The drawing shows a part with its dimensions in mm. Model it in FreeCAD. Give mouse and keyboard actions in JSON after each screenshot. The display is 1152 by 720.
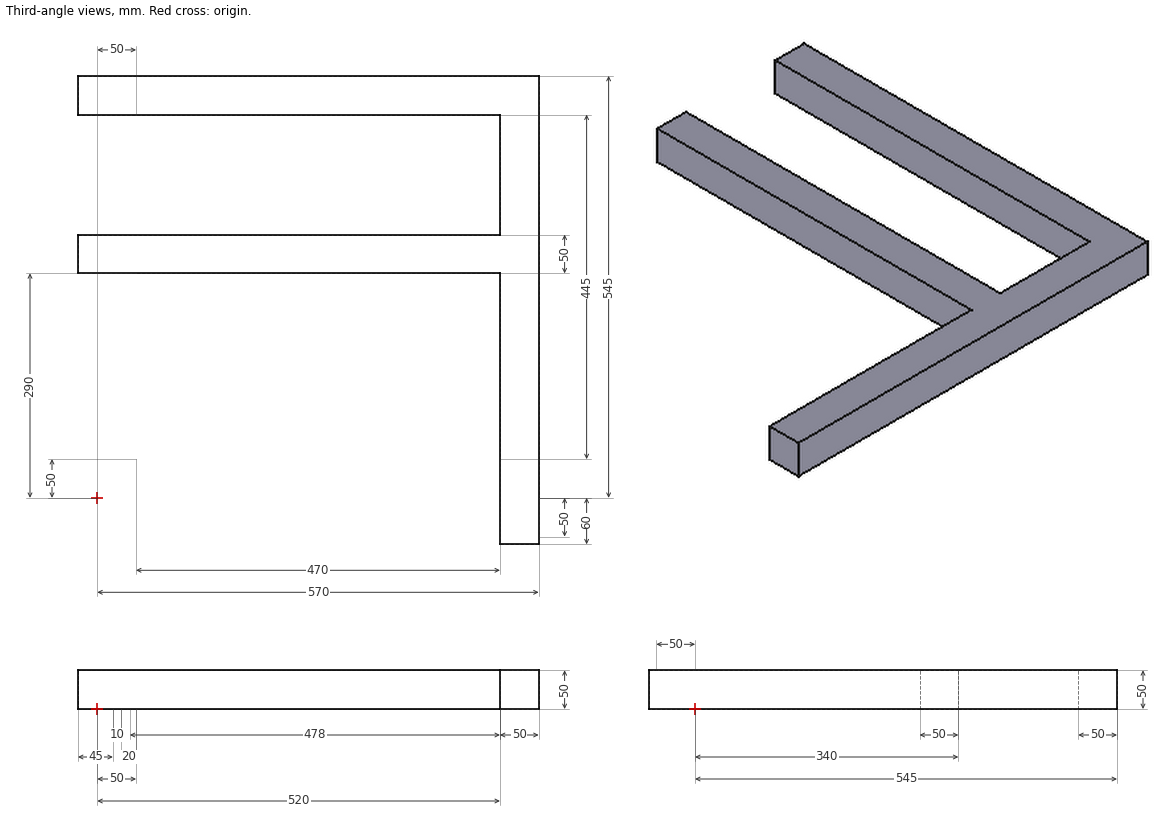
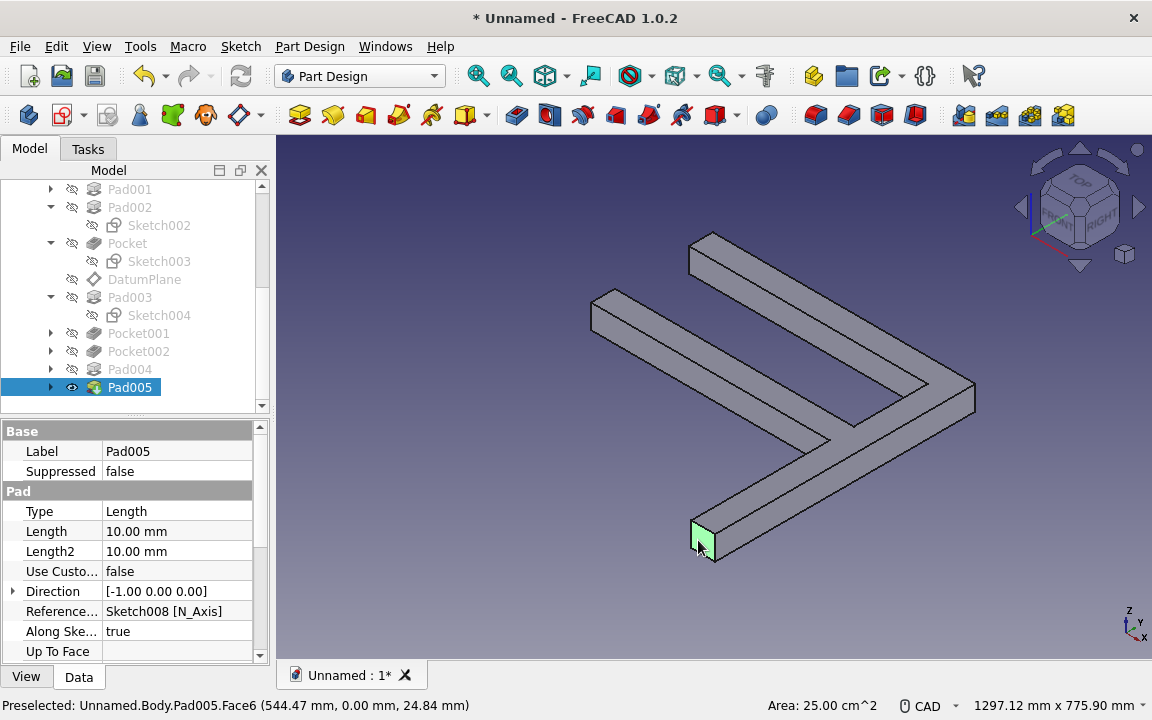
{"action": "left_click", "coordinate": [62, 116]}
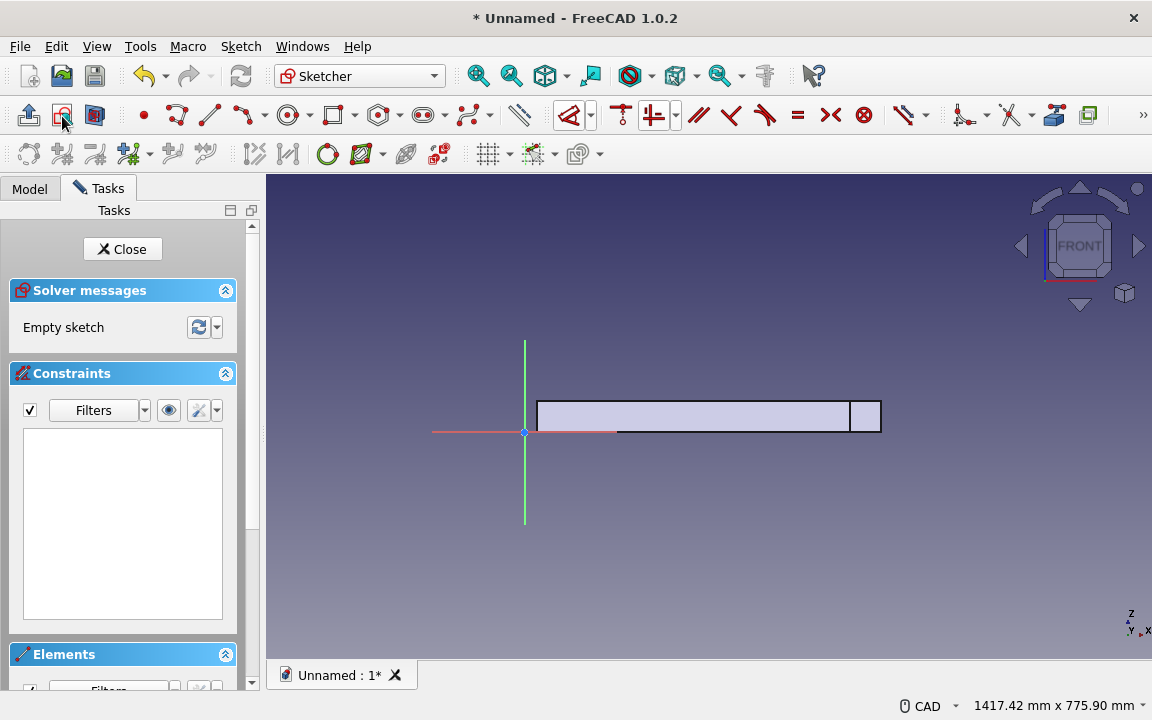
{"action": "scroll", "coordinate": [893, 416], "scroll_direction": "up", "scroll_amount": 11}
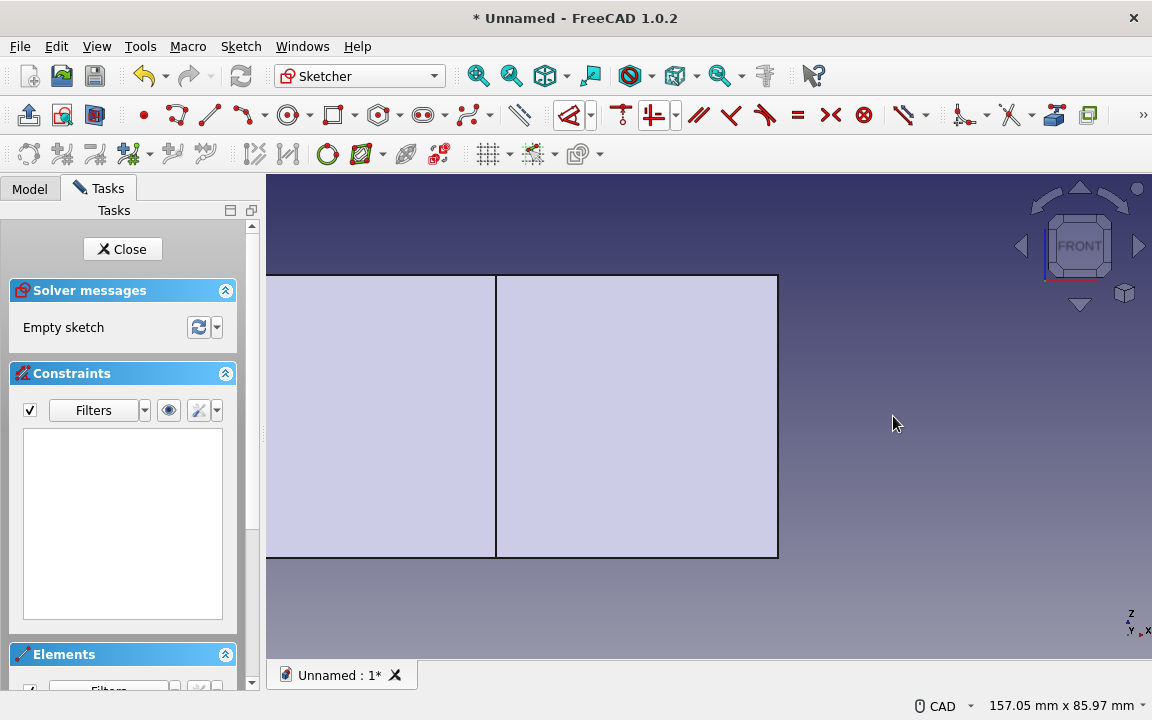
{"action": "key", "text": "g r"}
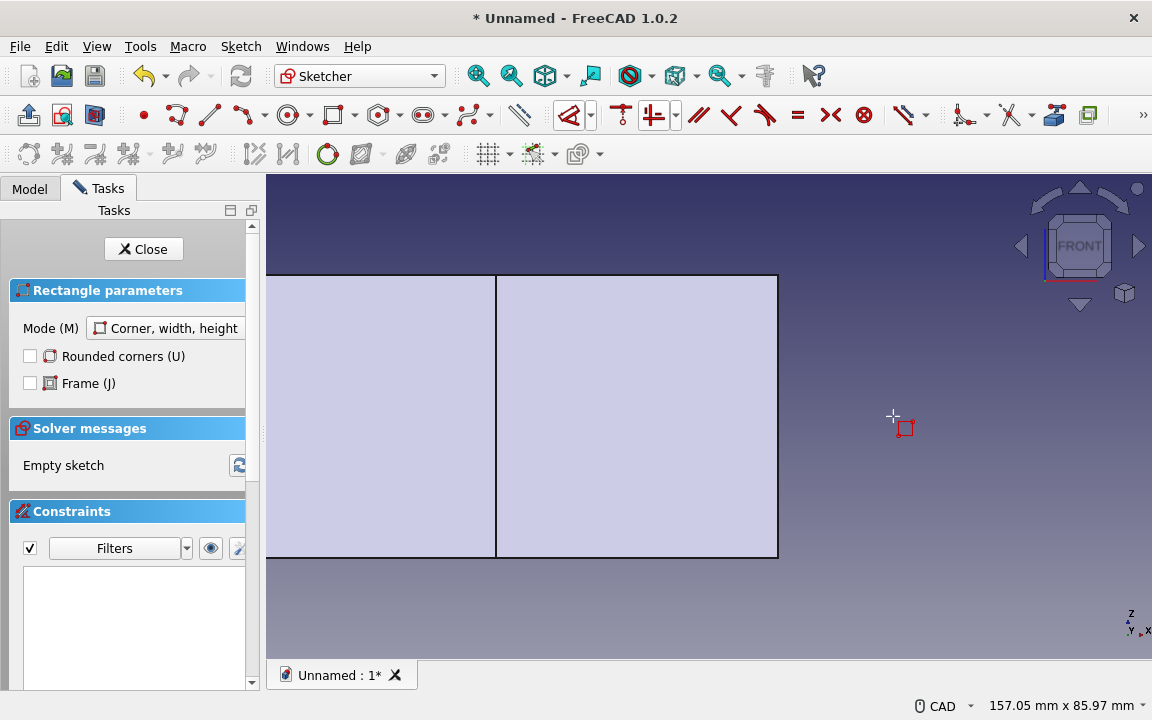
{"action": "left_click", "coordinate": [496, 275]}
{"action": "left_click", "coordinate": [778, 558]}
{"action": "key", "text": "Escape"}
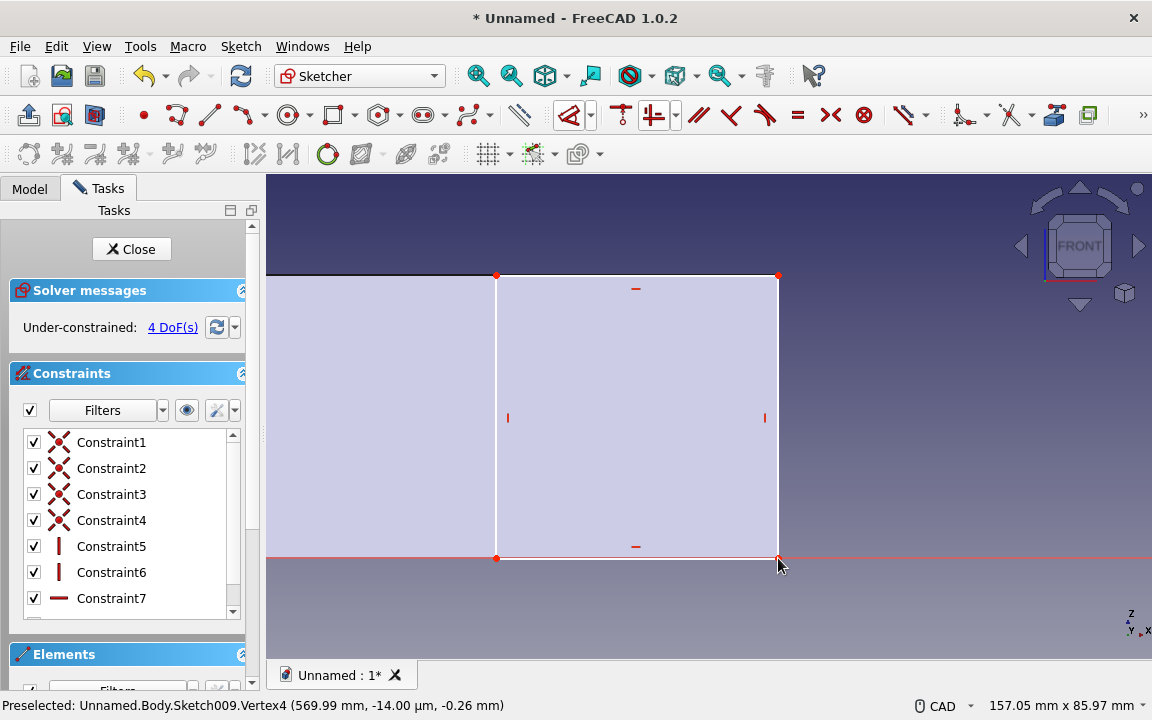
{"action": "left_click", "coordinate": [496, 559]}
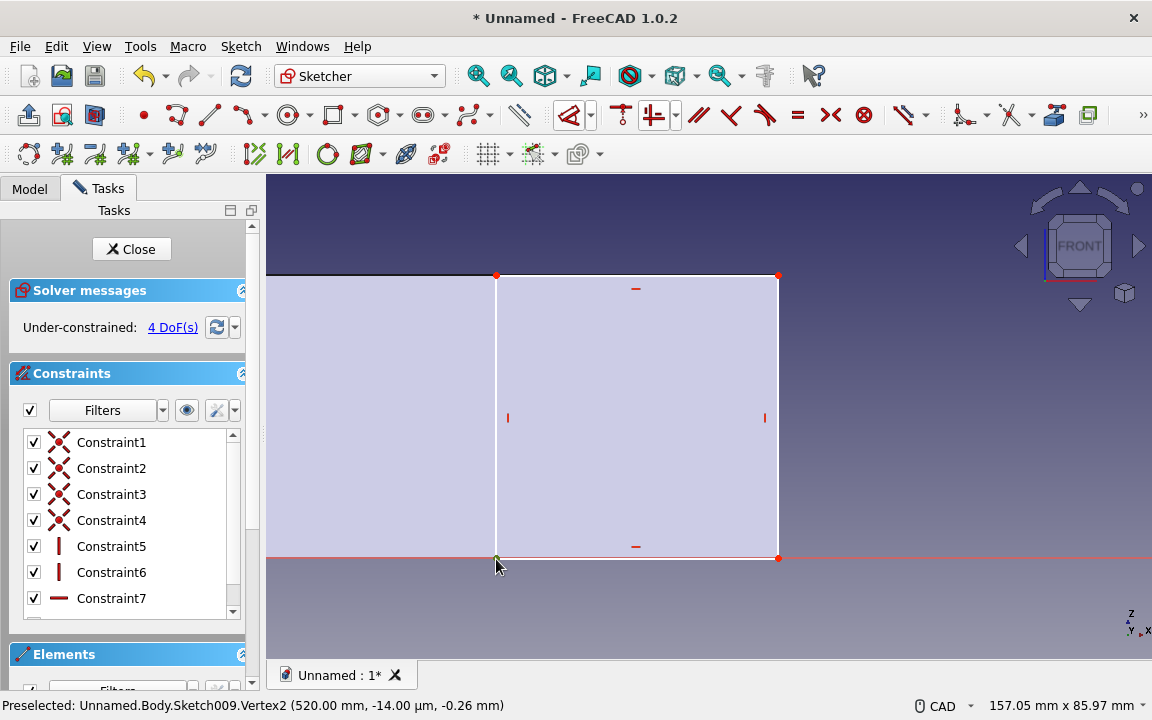
{"action": "left_click", "coordinate": [344, 558]}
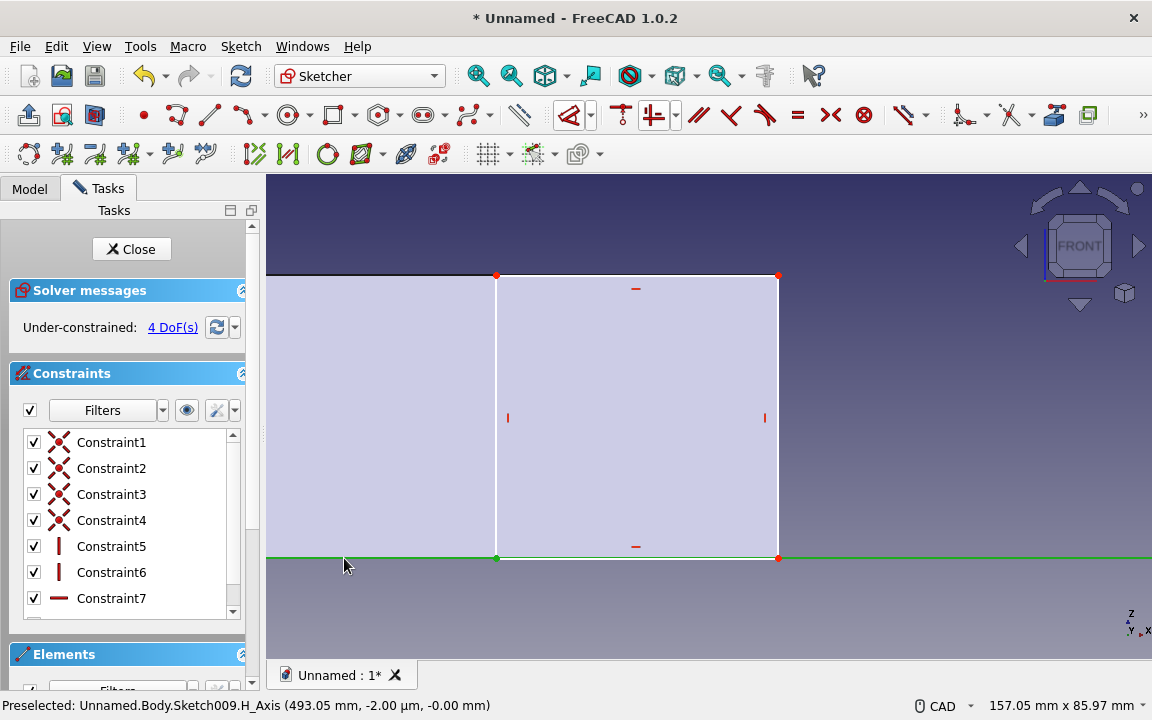
{"action": "key", "text": "c"}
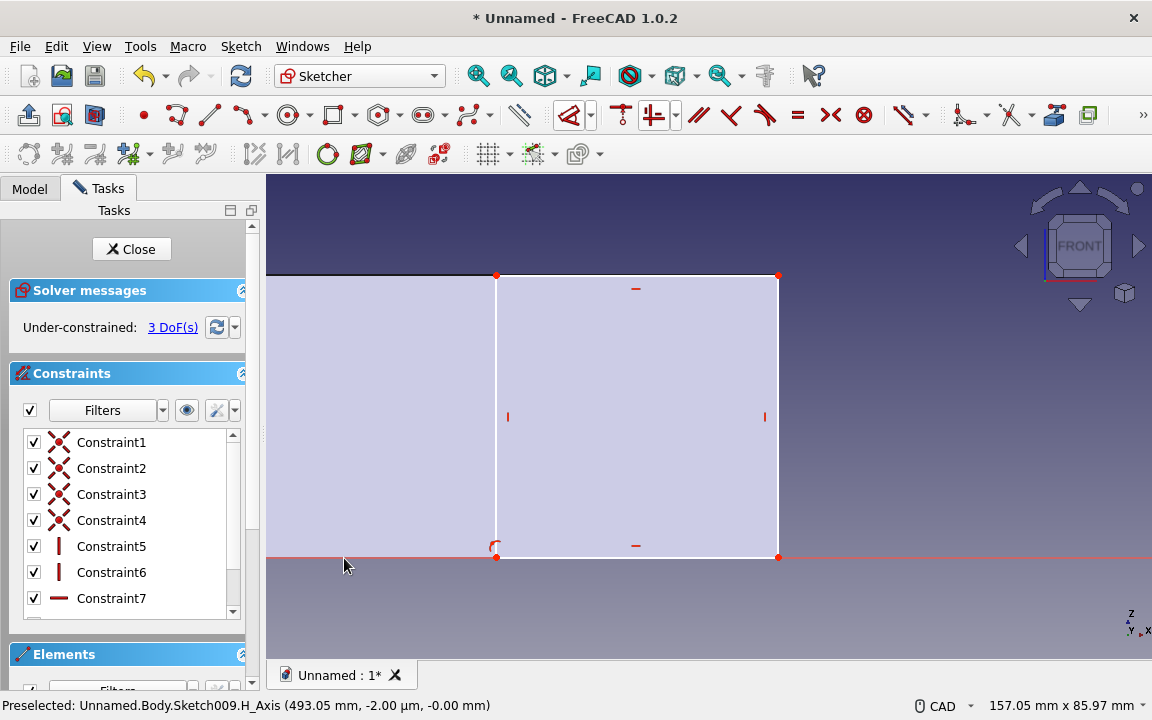
{"action": "left_click", "coordinate": [496, 360]}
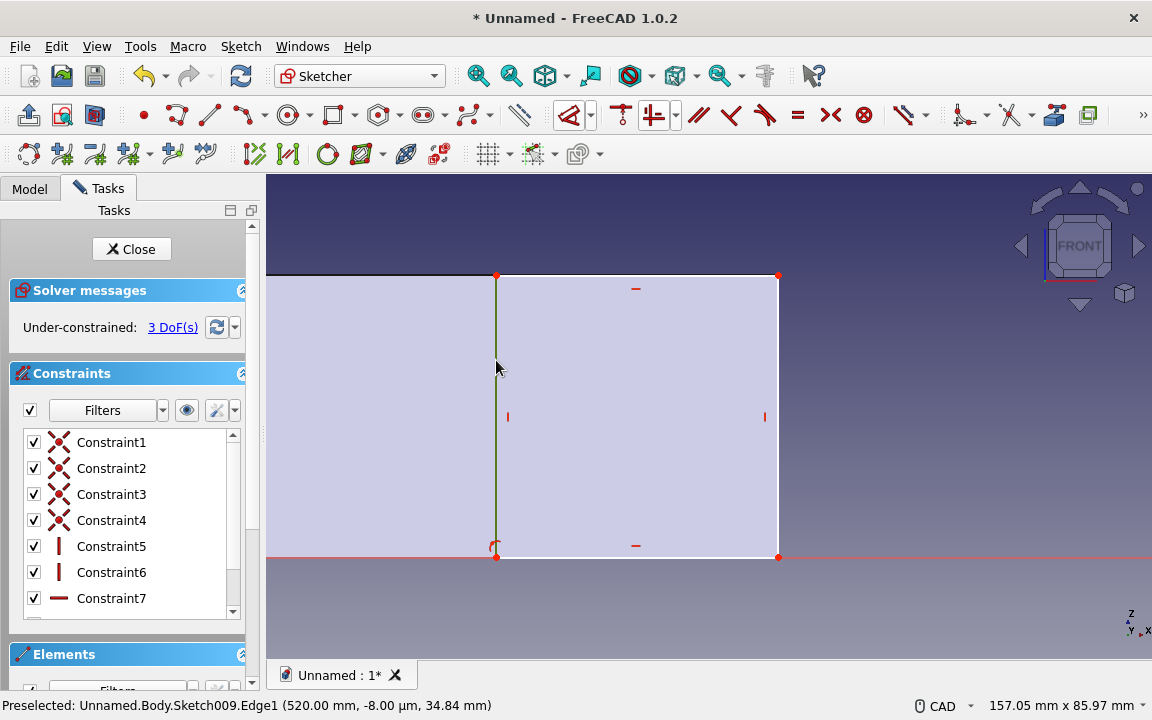
{"action": "key", "text": "i"}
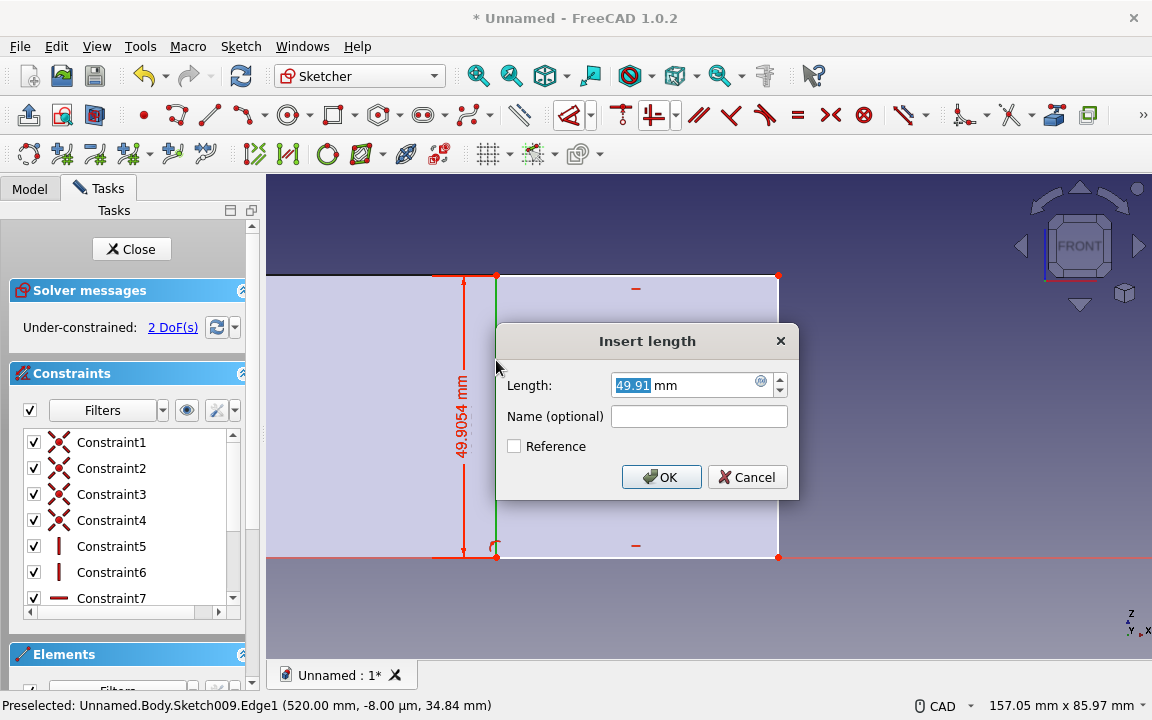
{"action": "type", "text": "50"}
{"action": "key", "text": "Return"}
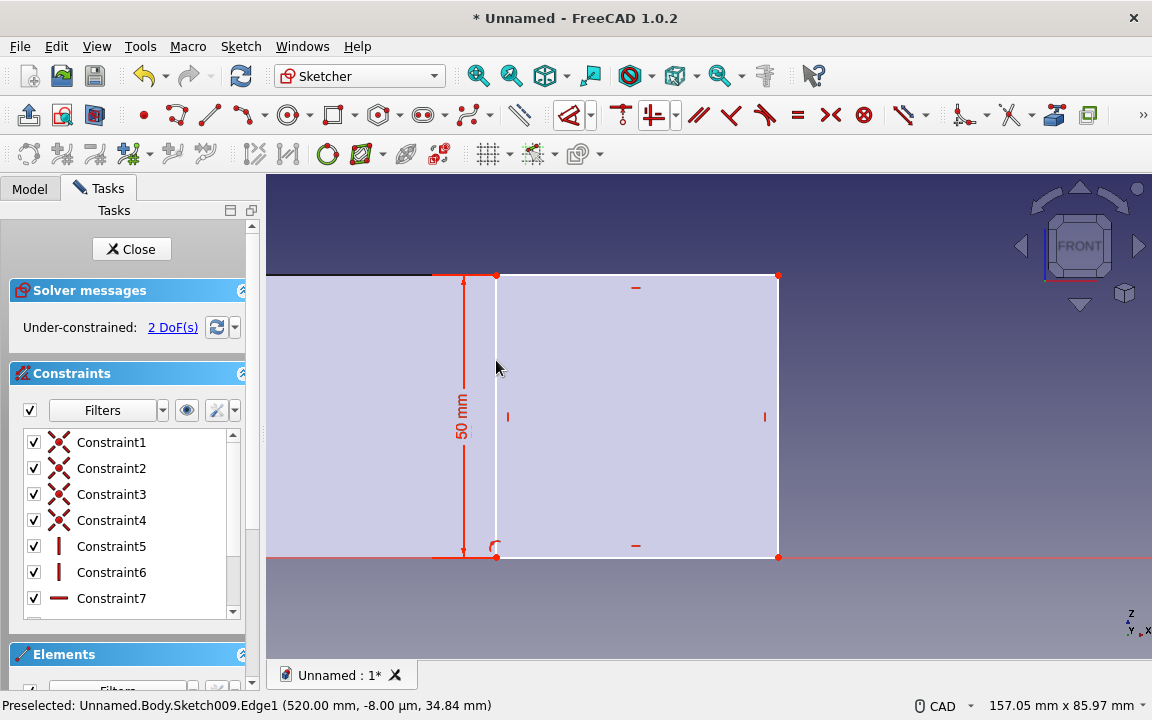
{"action": "left_click", "coordinate": [581, 558]}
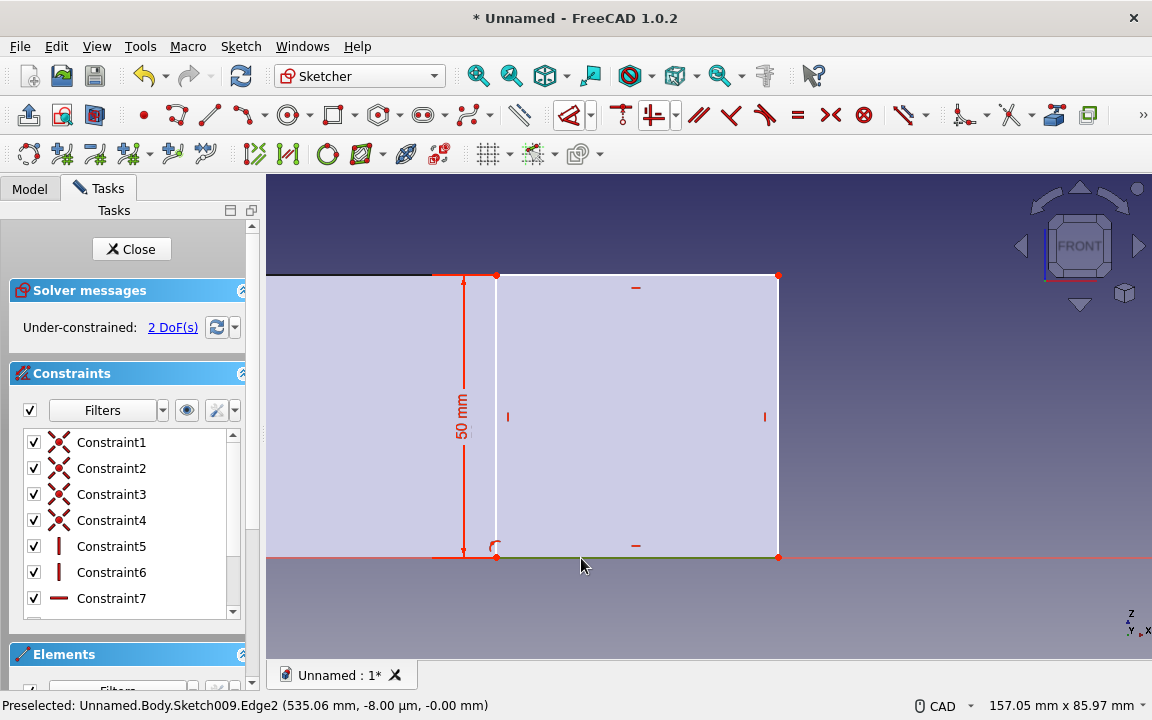
{"action": "left_click", "coordinate": [590, 116]}